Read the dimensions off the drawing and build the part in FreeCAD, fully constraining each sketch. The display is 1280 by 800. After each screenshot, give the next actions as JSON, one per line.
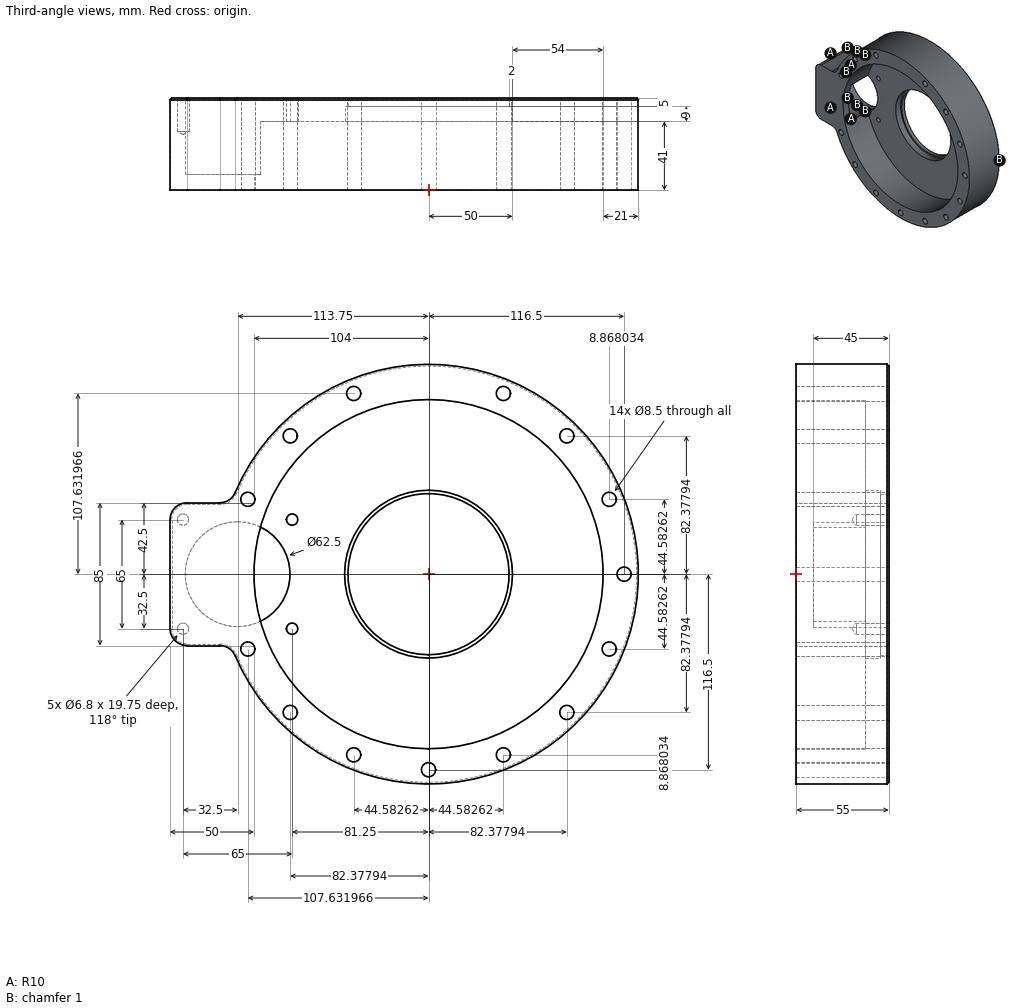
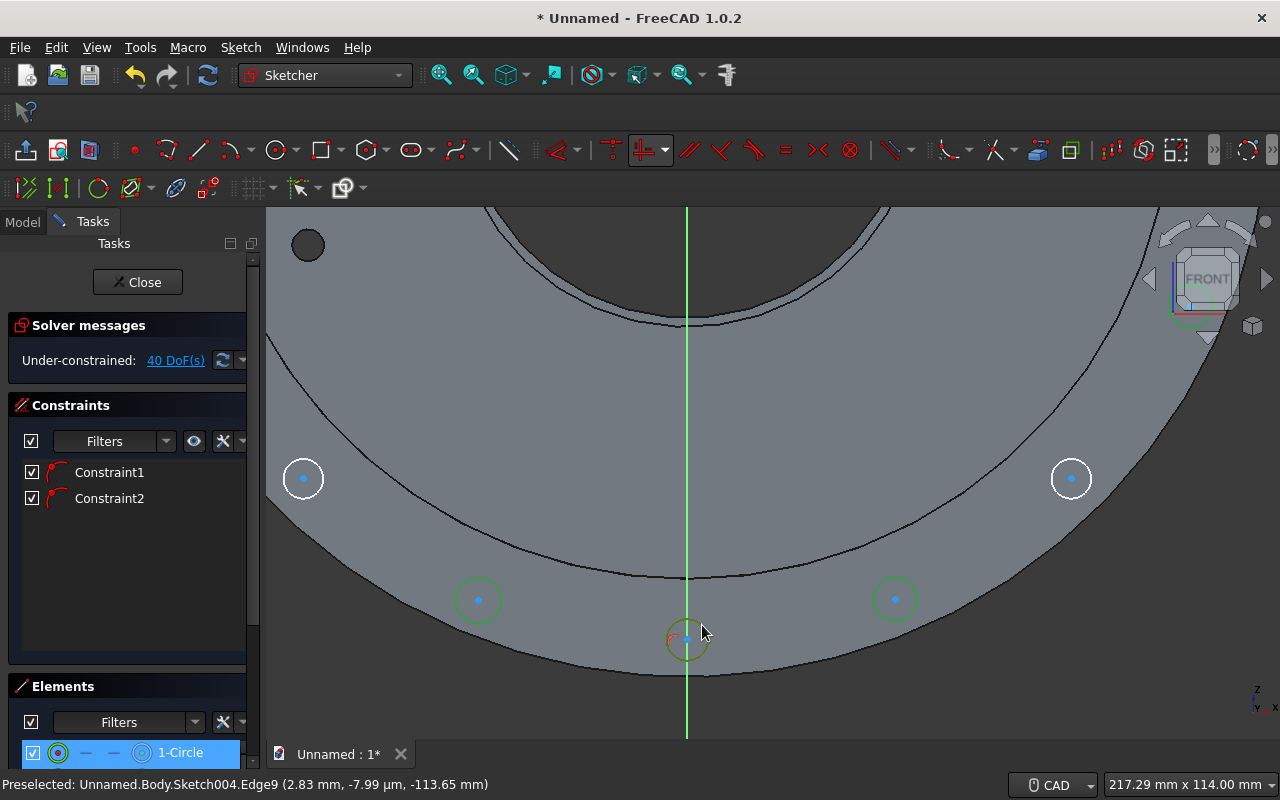
{"action": "left_click", "coordinate": [1085, 465]}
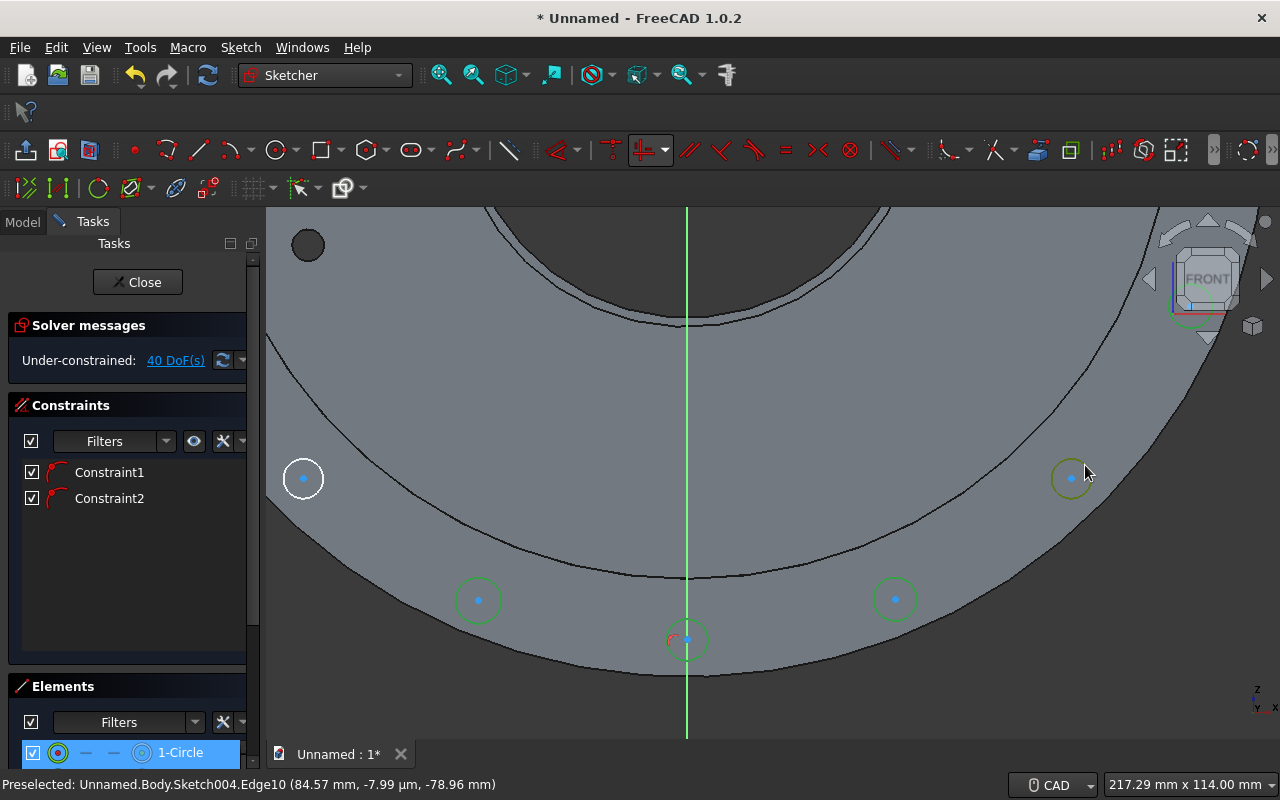
{"action": "left_click", "coordinate": [317, 465]}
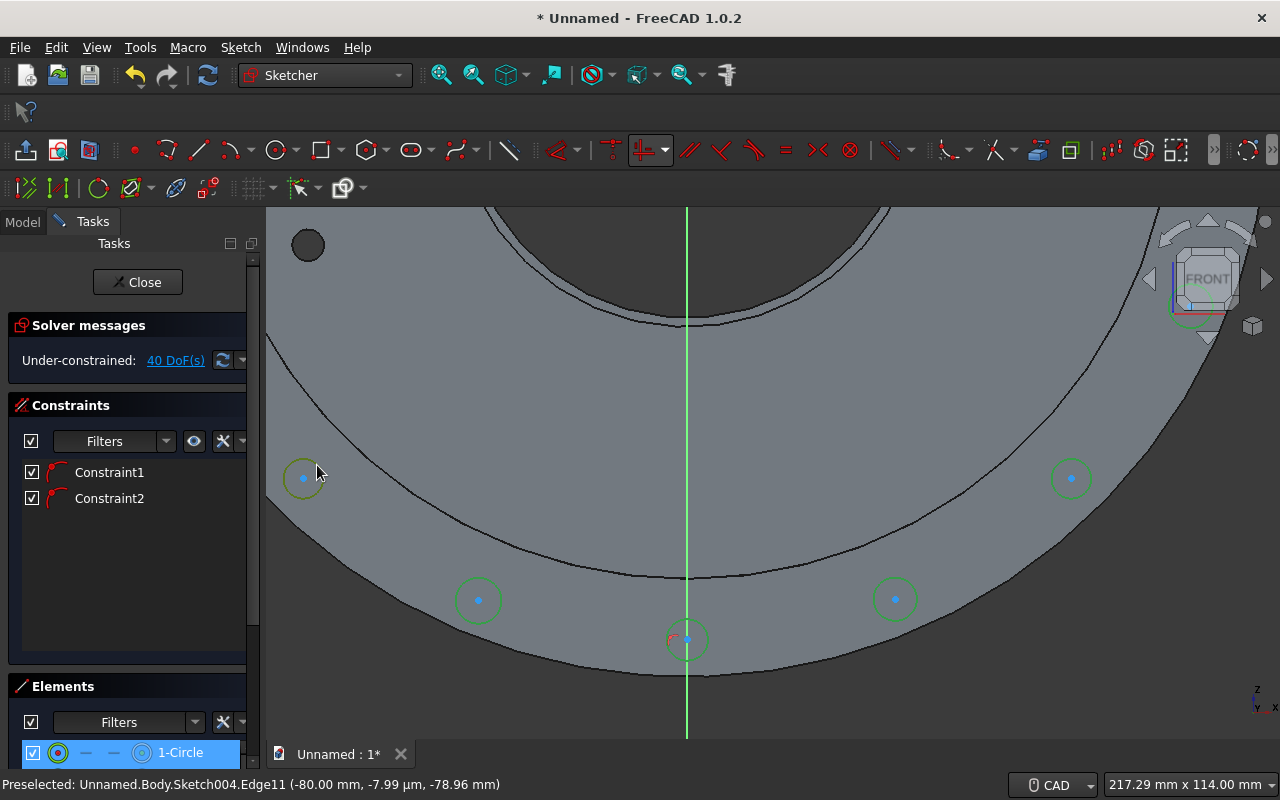
{"action": "scroll", "coordinate": [703, 628], "scroll_direction": "down", "scroll_amount": 6}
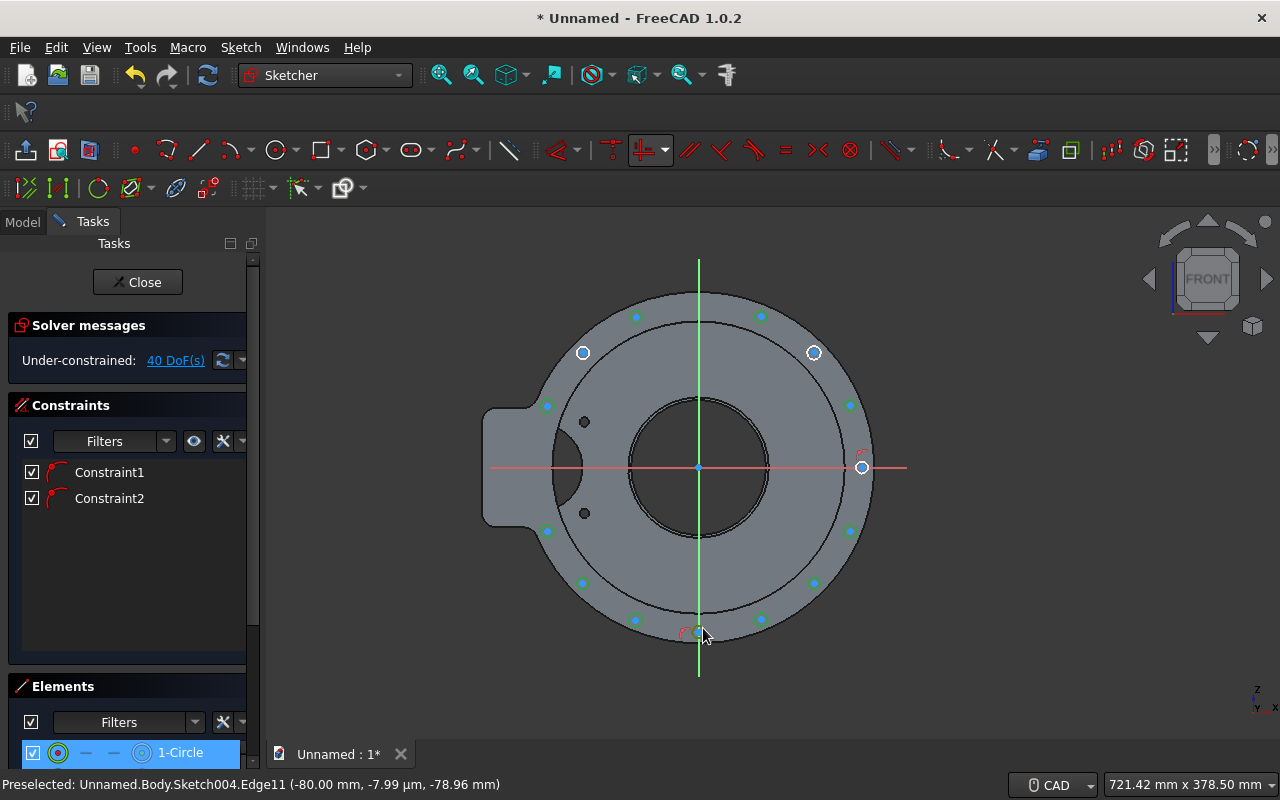
{"action": "scroll", "coordinate": [819, 348], "scroll_direction": "up", "scroll_amount": 4}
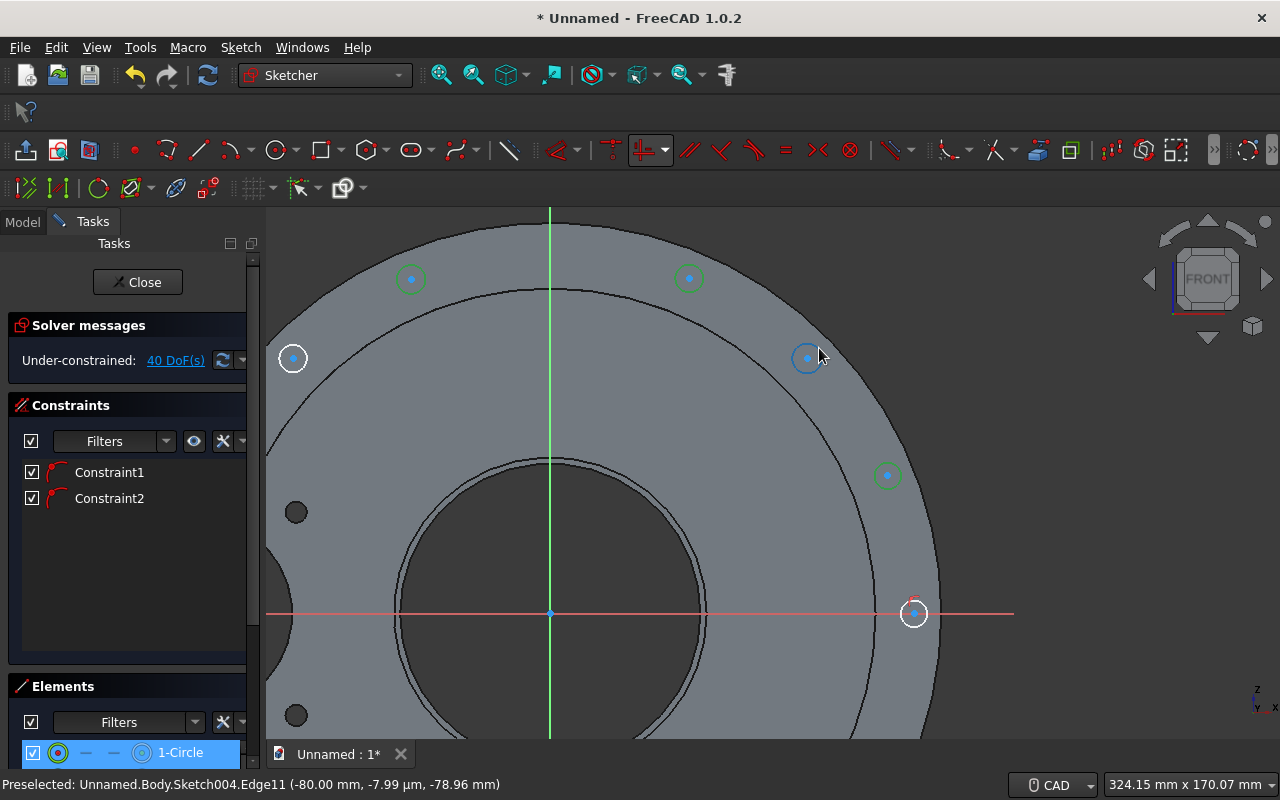
{"action": "left_click", "coordinate": [818, 348]}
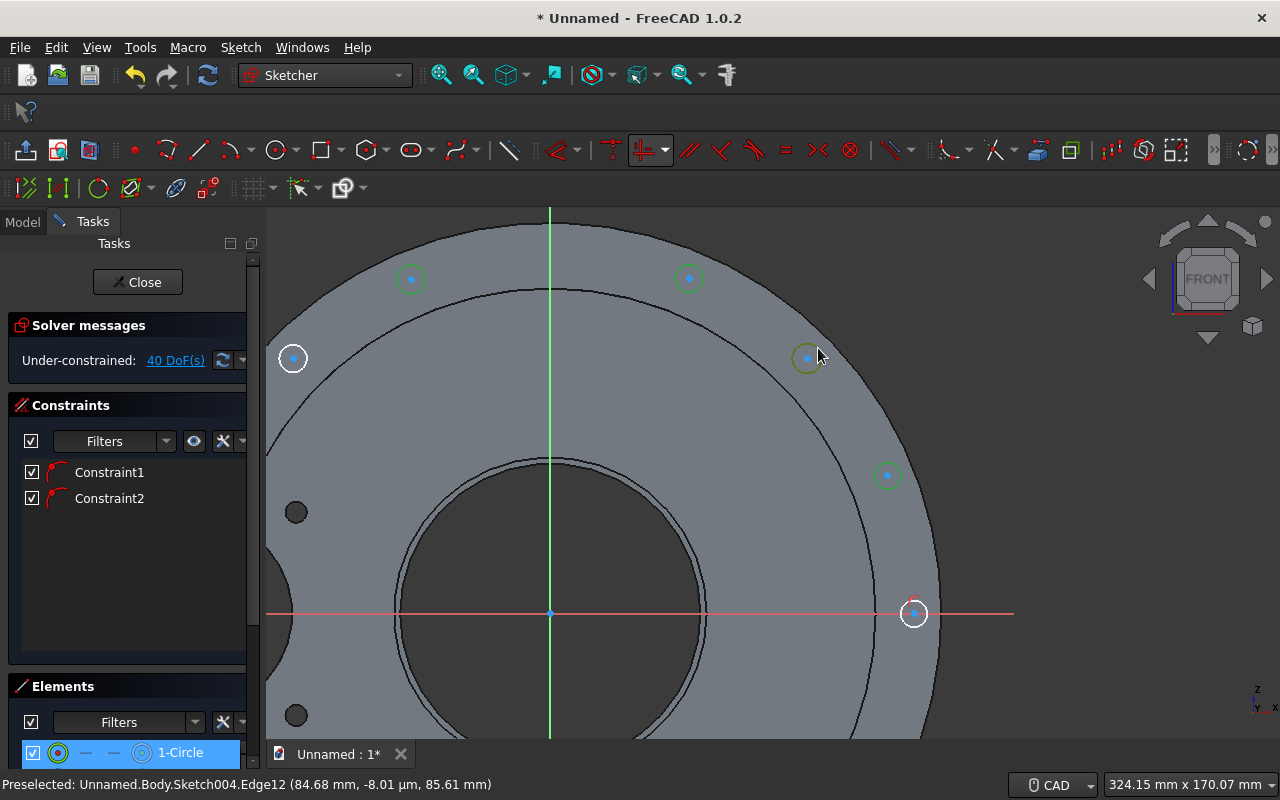
{"action": "left_click", "coordinate": [303, 349]}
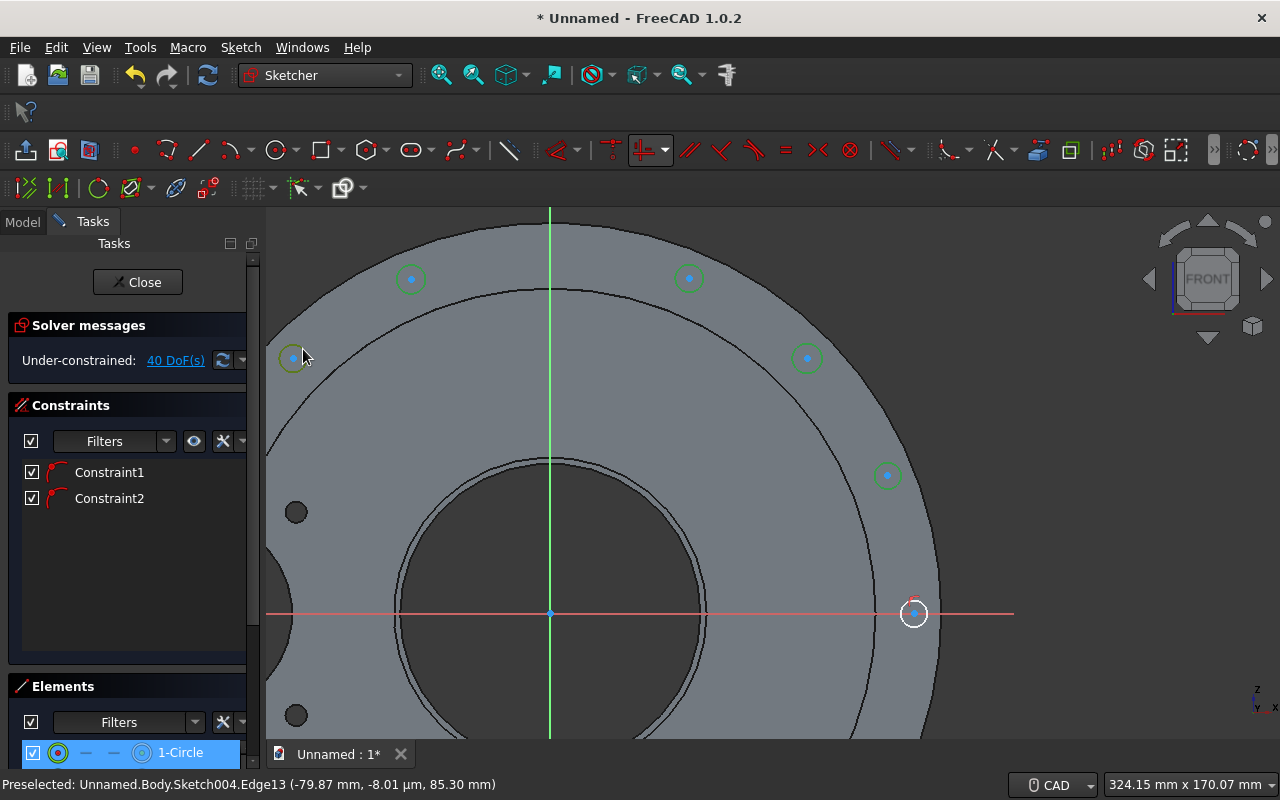
{"action": "scroll", "coordinate": [923, 604], "scroll_direction": "up", "scroll_amount": 2}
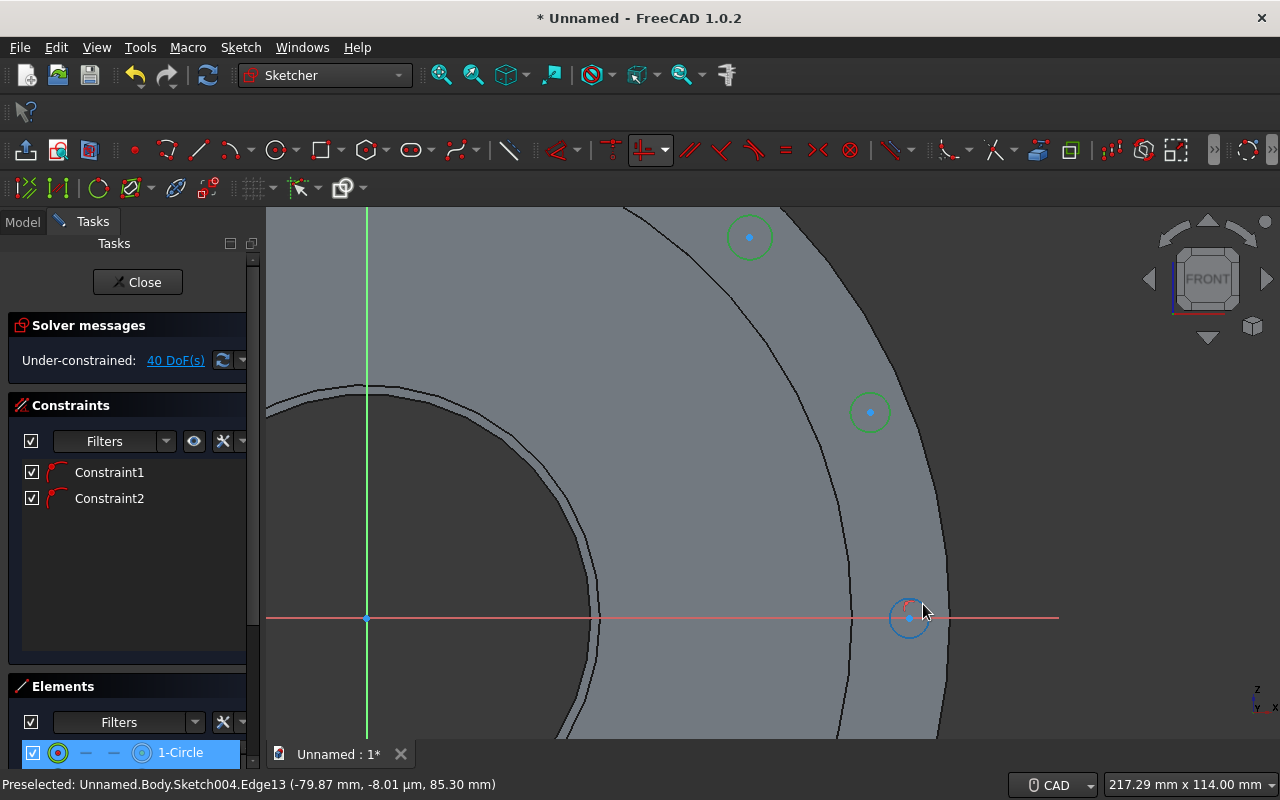
{"action": "left_click", "coordinate": [923, 604]}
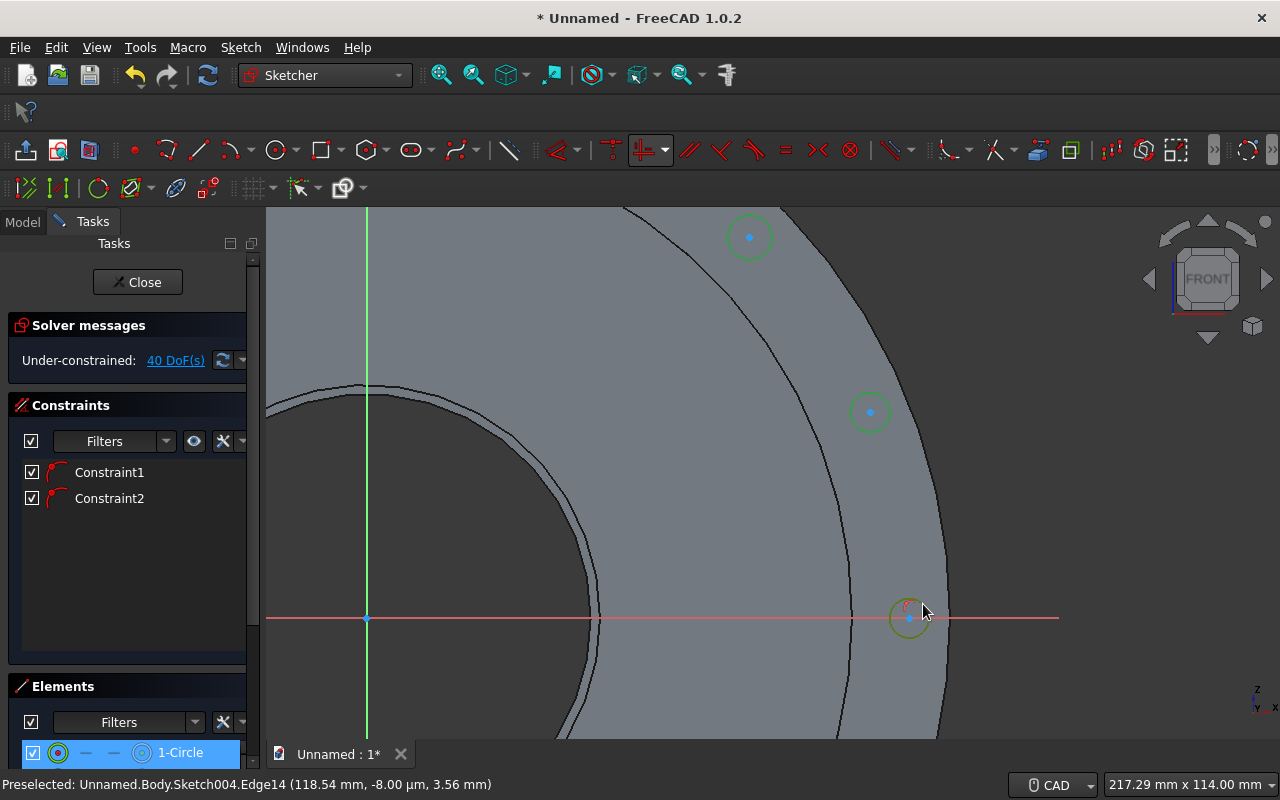
{"action": "left_click", "coordinate": [786, 150]}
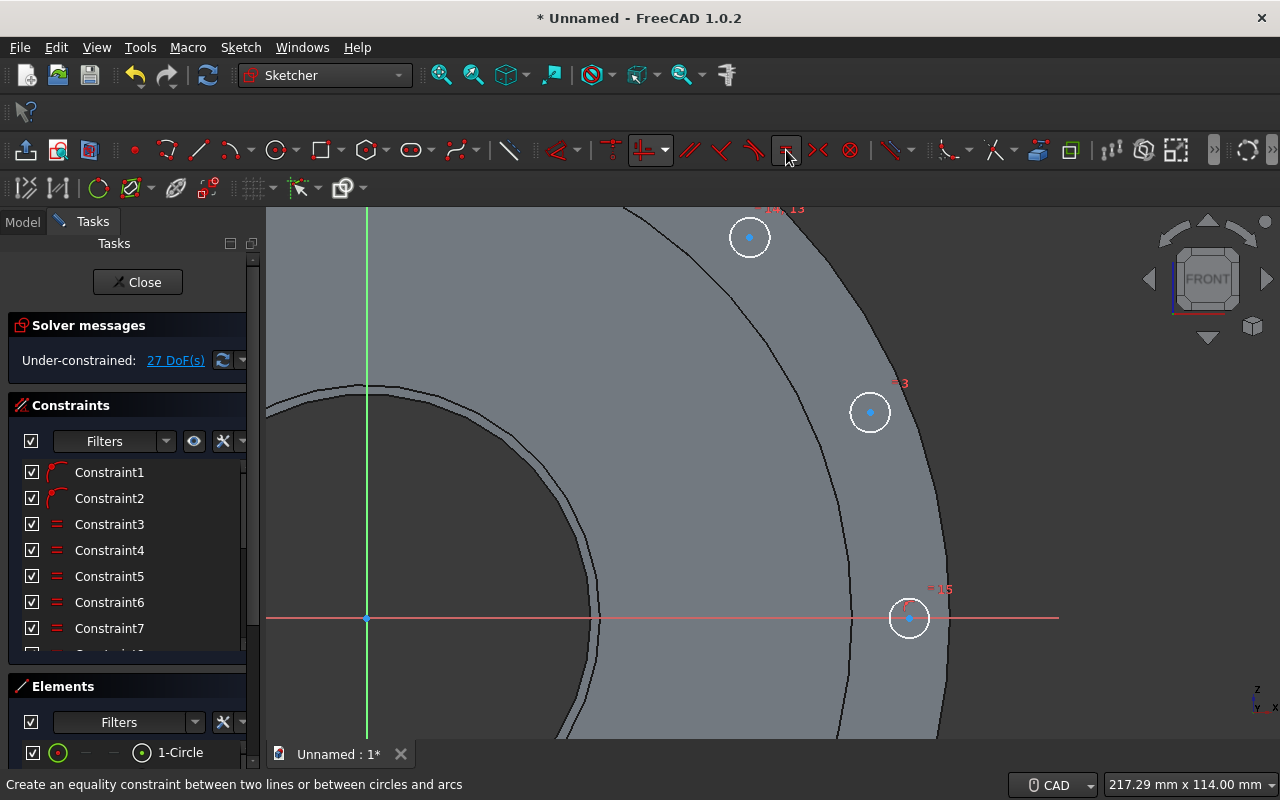
{"action": "left_click", "coordinate": [870, 413]}